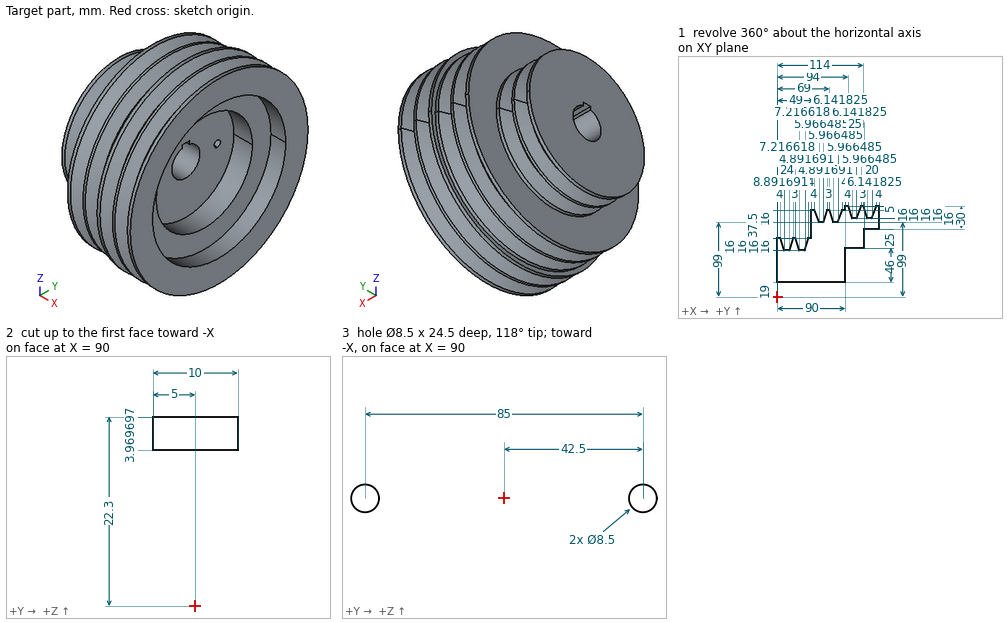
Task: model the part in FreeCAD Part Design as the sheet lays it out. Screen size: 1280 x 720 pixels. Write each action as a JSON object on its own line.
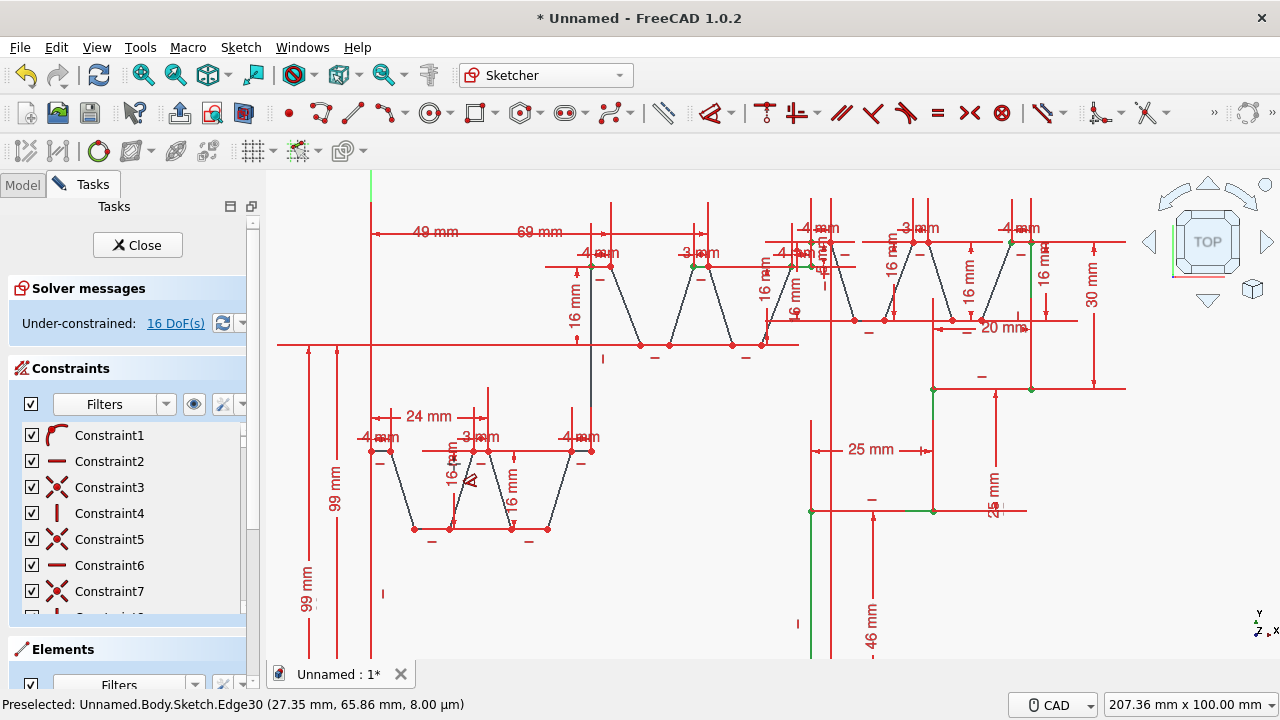
{"action": "left_click", "coordinate": [467, 475]}
{"action": "left_click", "coordinate": [392, 517]}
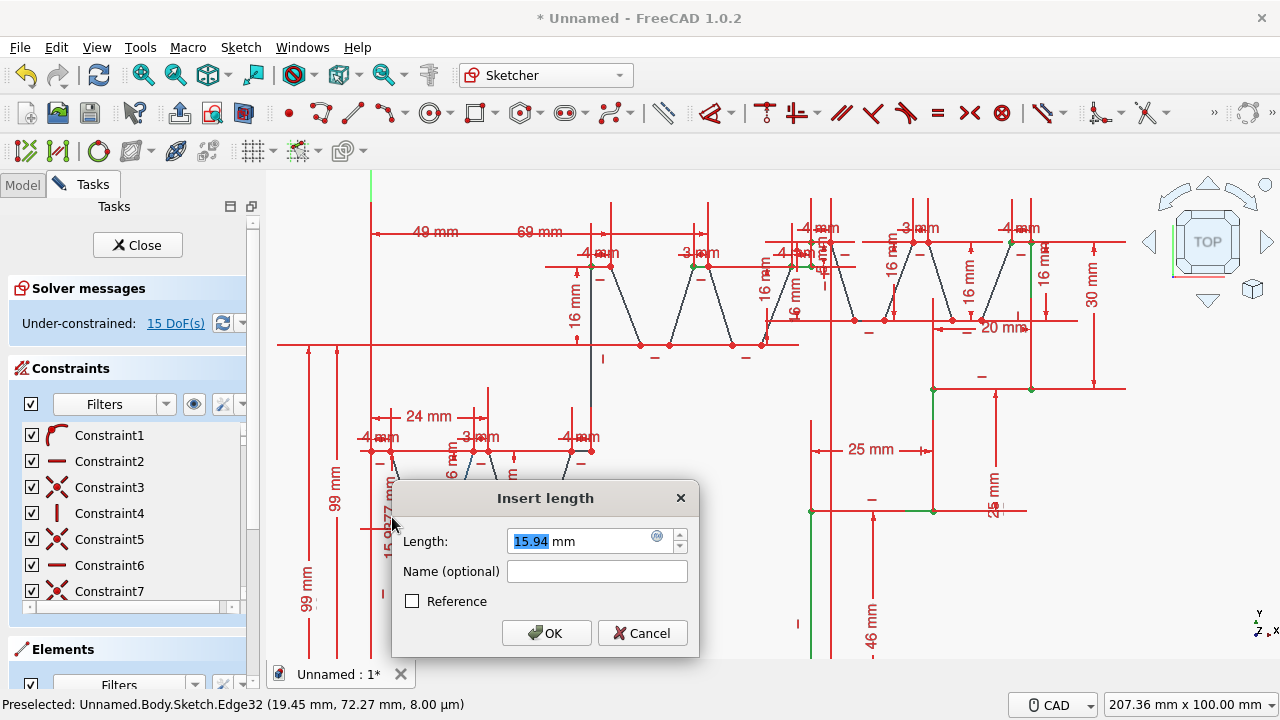
{"action": "type", "text": "16"}
{"action": "key", "text": "Return"}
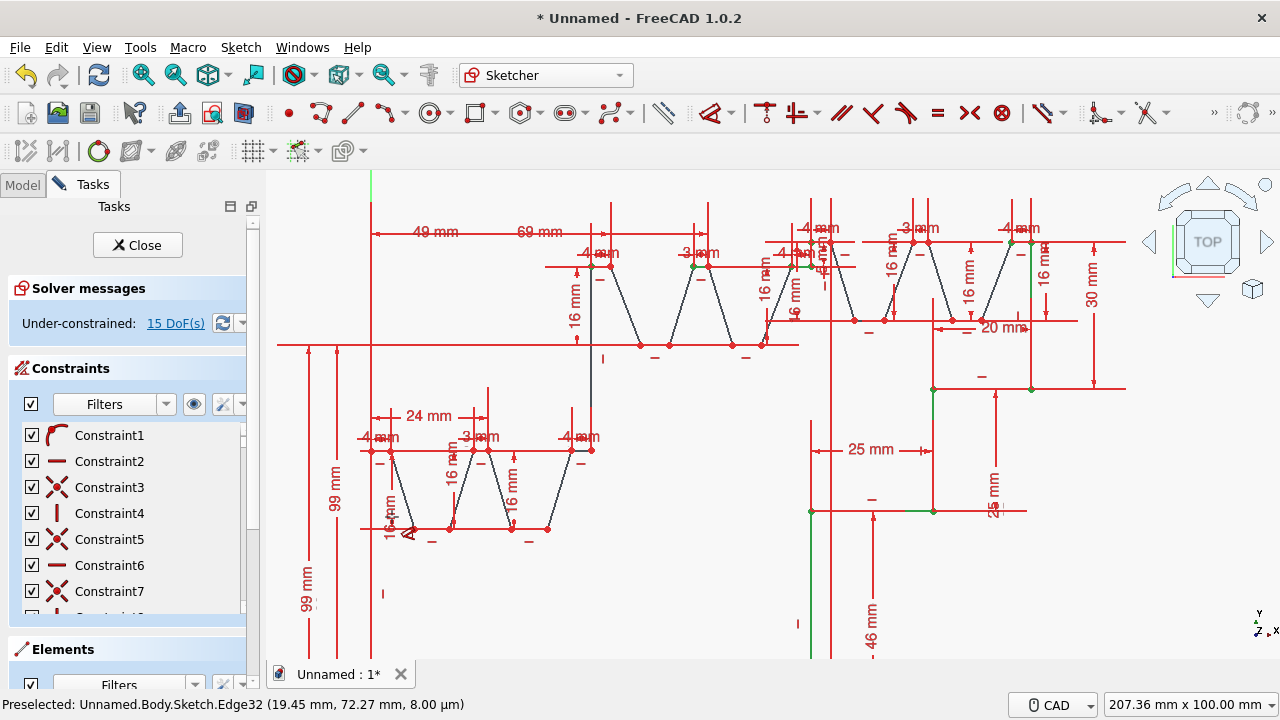
{"action": "left_click", "coordinate": [407, 506]}
{"action": "left_click", "coordinate": [357, 463]}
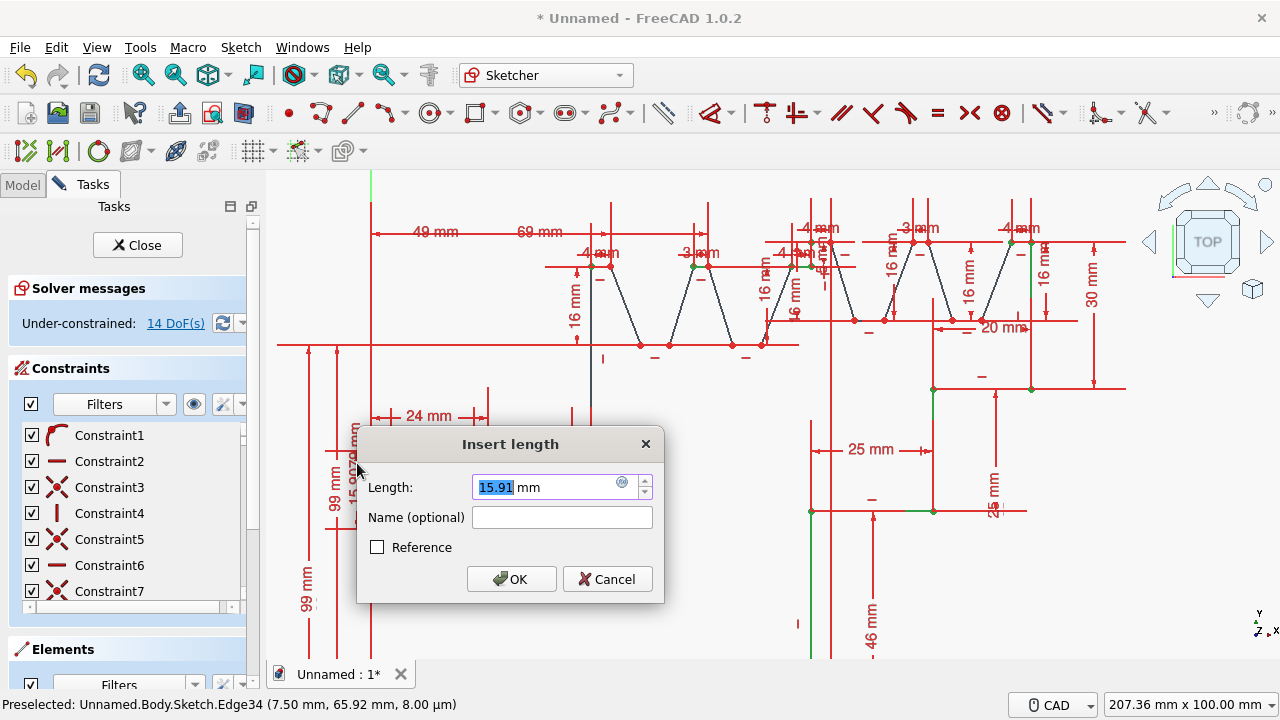
{"action": "type", "text": "16"}
{"action": "key", "text": "Return"}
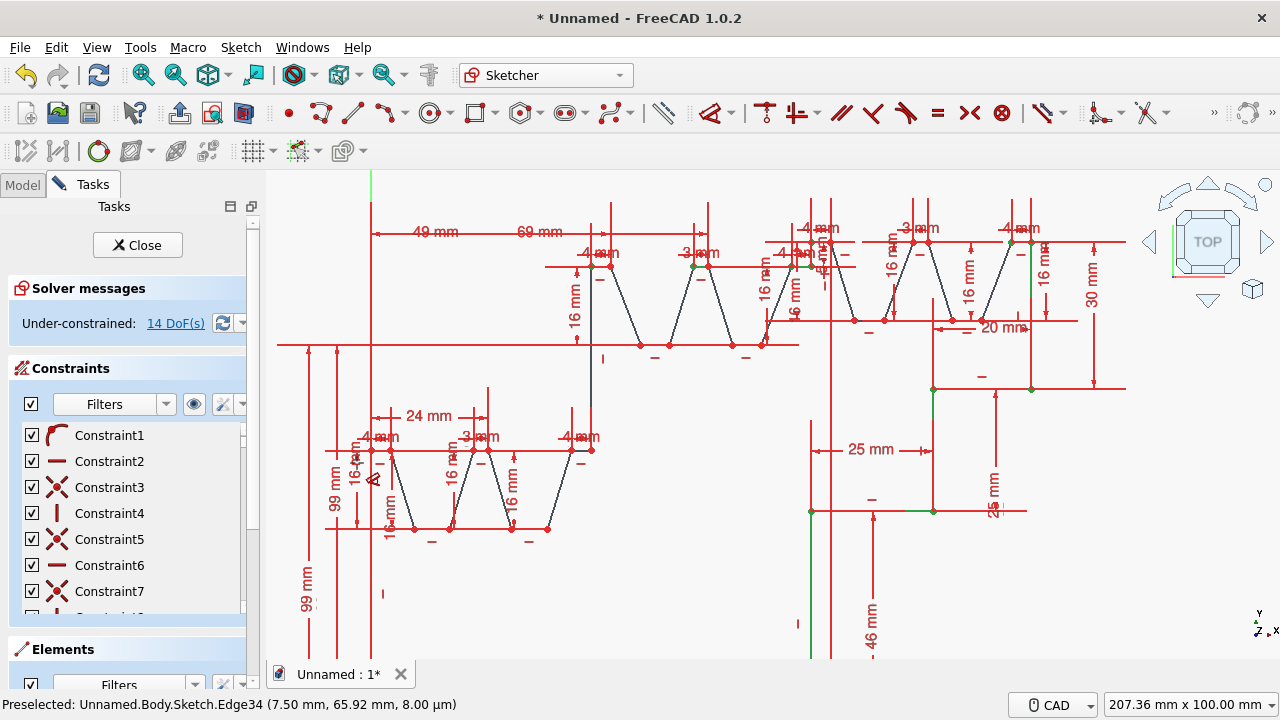
{"action": "left_click", "coordinate": [591, 322]}
{"action": "left_click", "coordinate": [557, 359]}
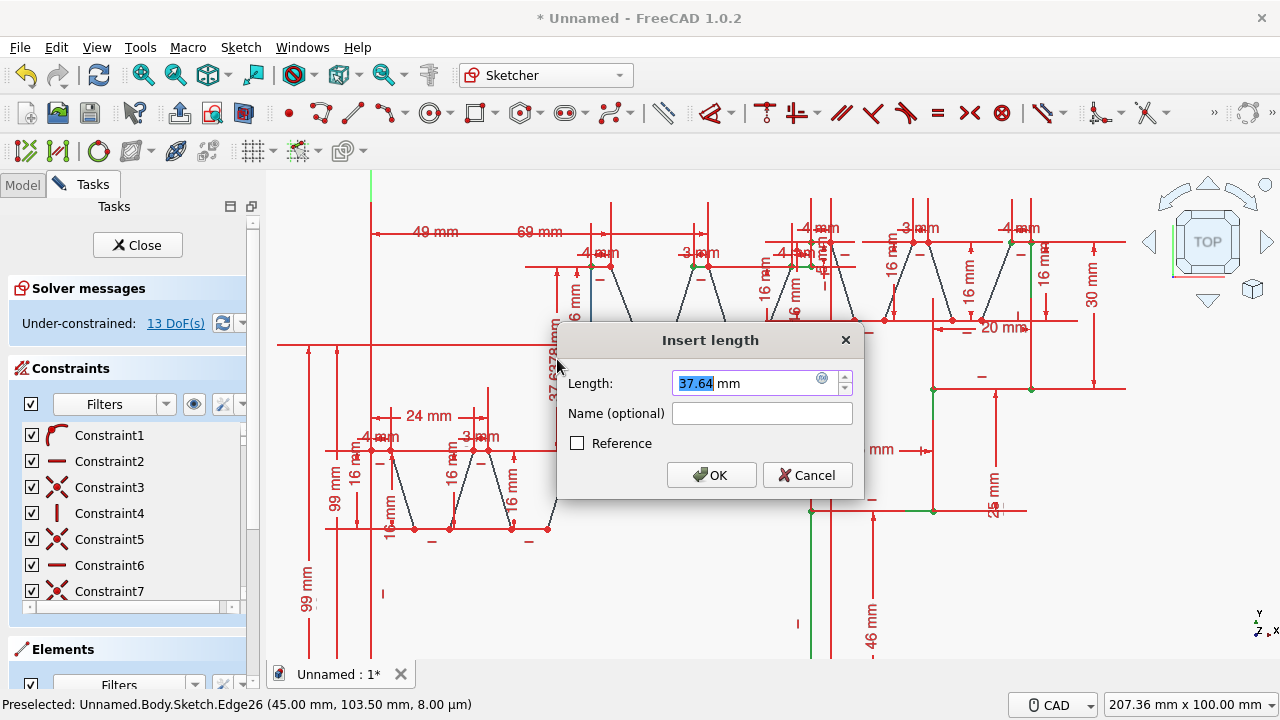
{"action": "type", "text": "37.5"}
{"action": "key", "text": "Return"}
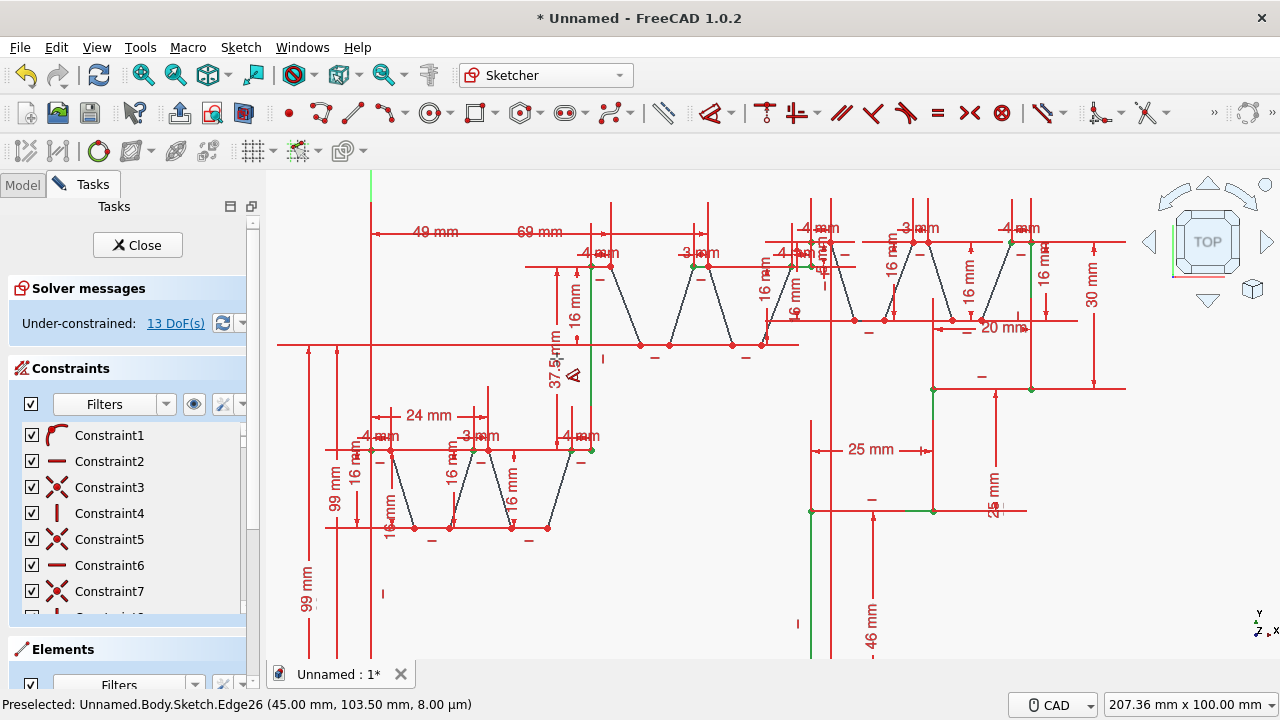
{"action": "left_click", "coordinate": [928, 242]}
{"action": "left_click", "coordinate": [650, 208]}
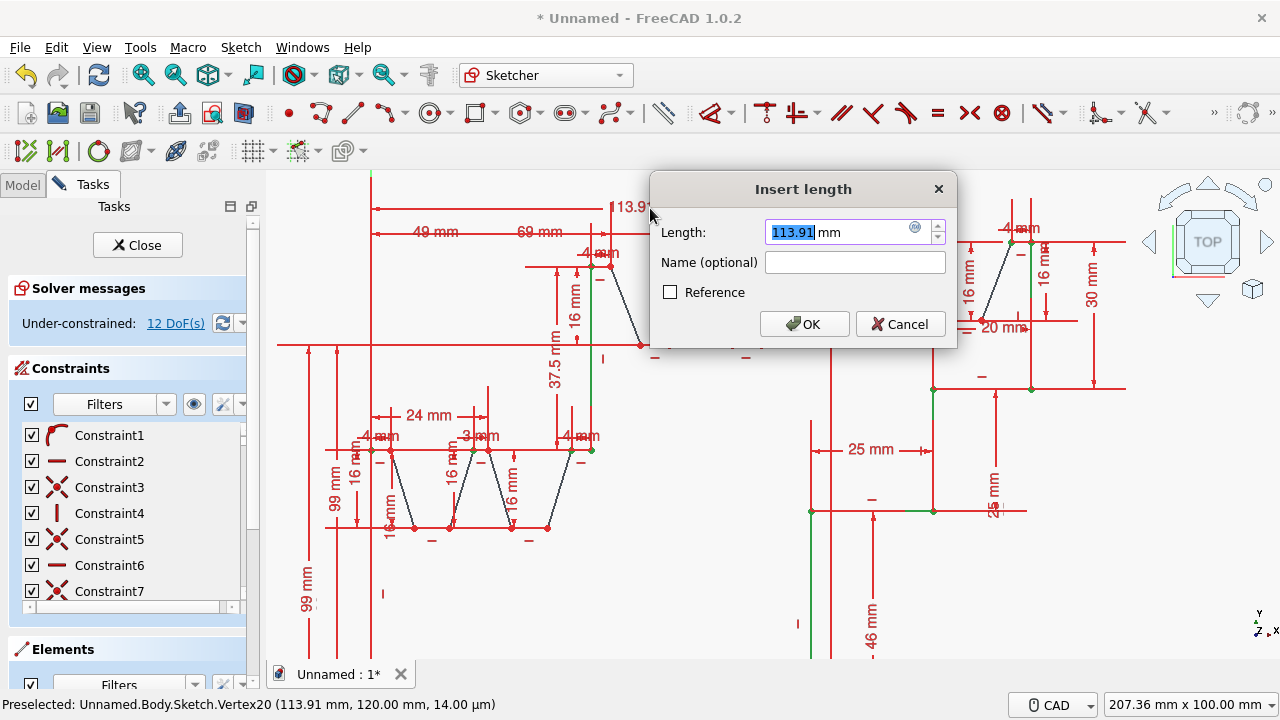
{"action": "type", "text": "114"}
{"action": "key", "text": "Return"}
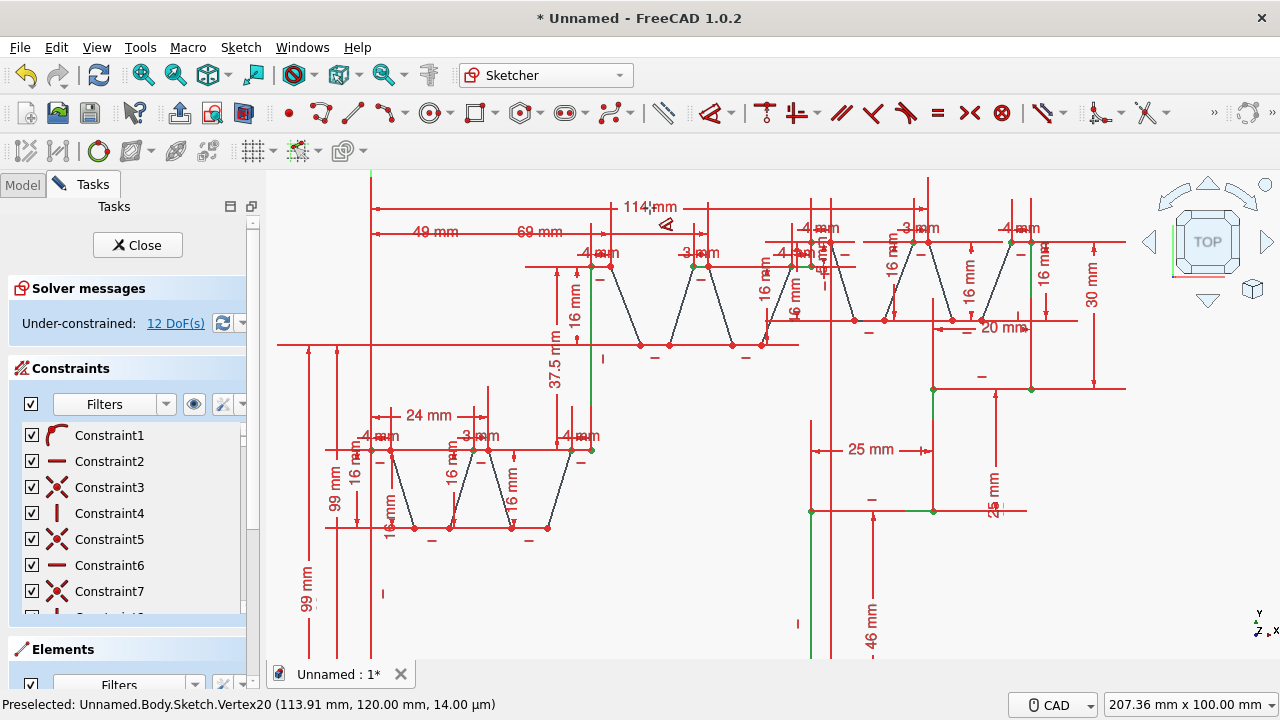
{"action": "scroll", "coordinate": [970, 321], "scroll_direction": "up", "scroll_amount": 2}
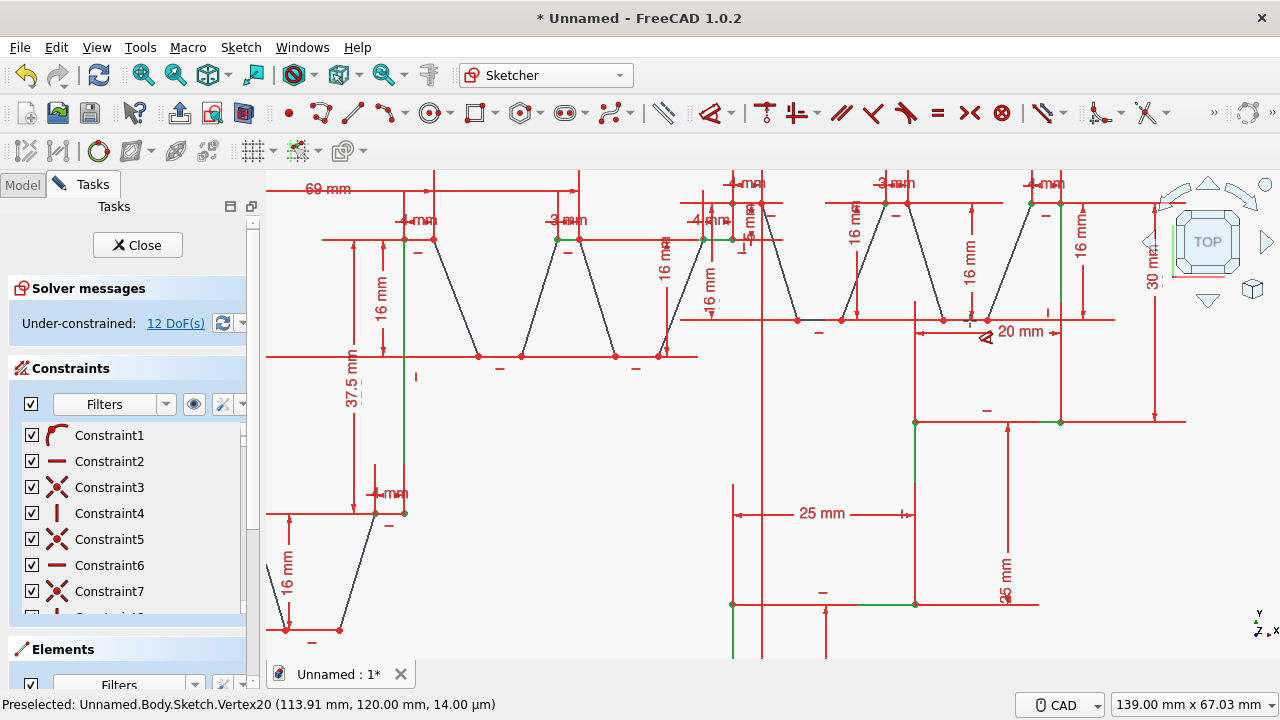
{"action": "left_click", "coordinate": [970, 320]}
{"action": "left_click", "coordinate": [965, 286]}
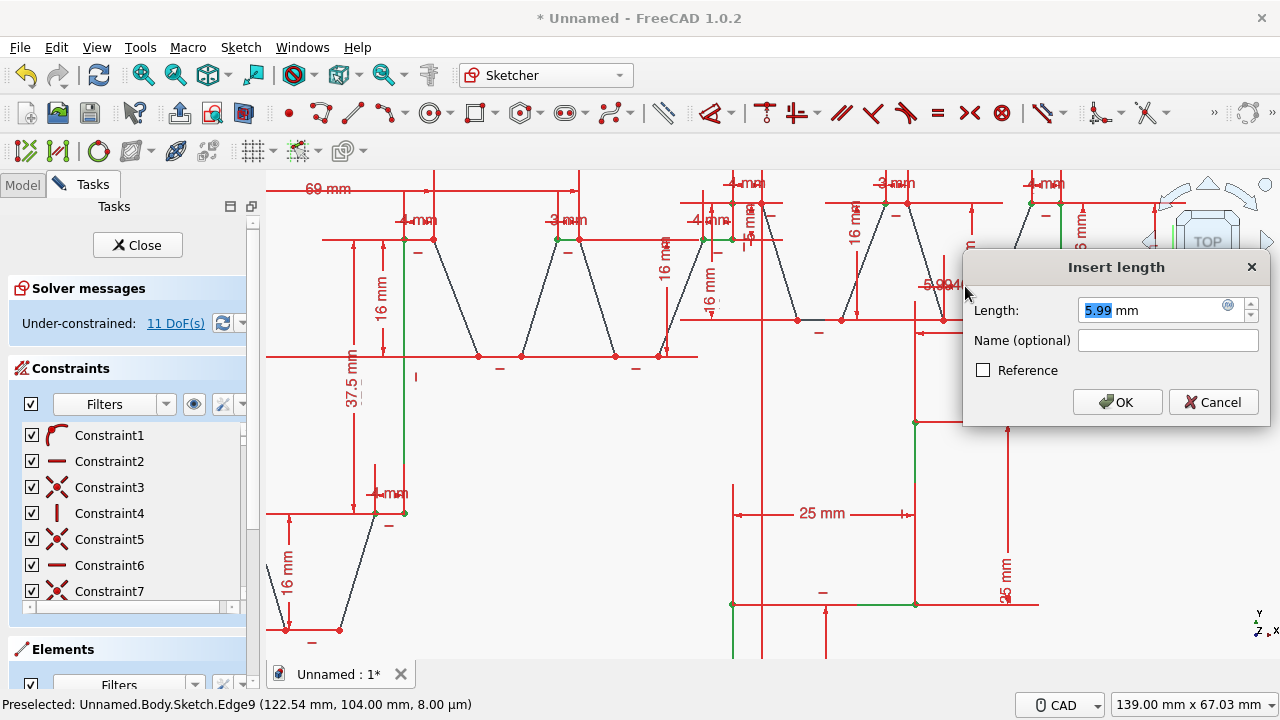
{"action": "type", "text": "5.966485"}
{"action": "key", "text": "Return"}